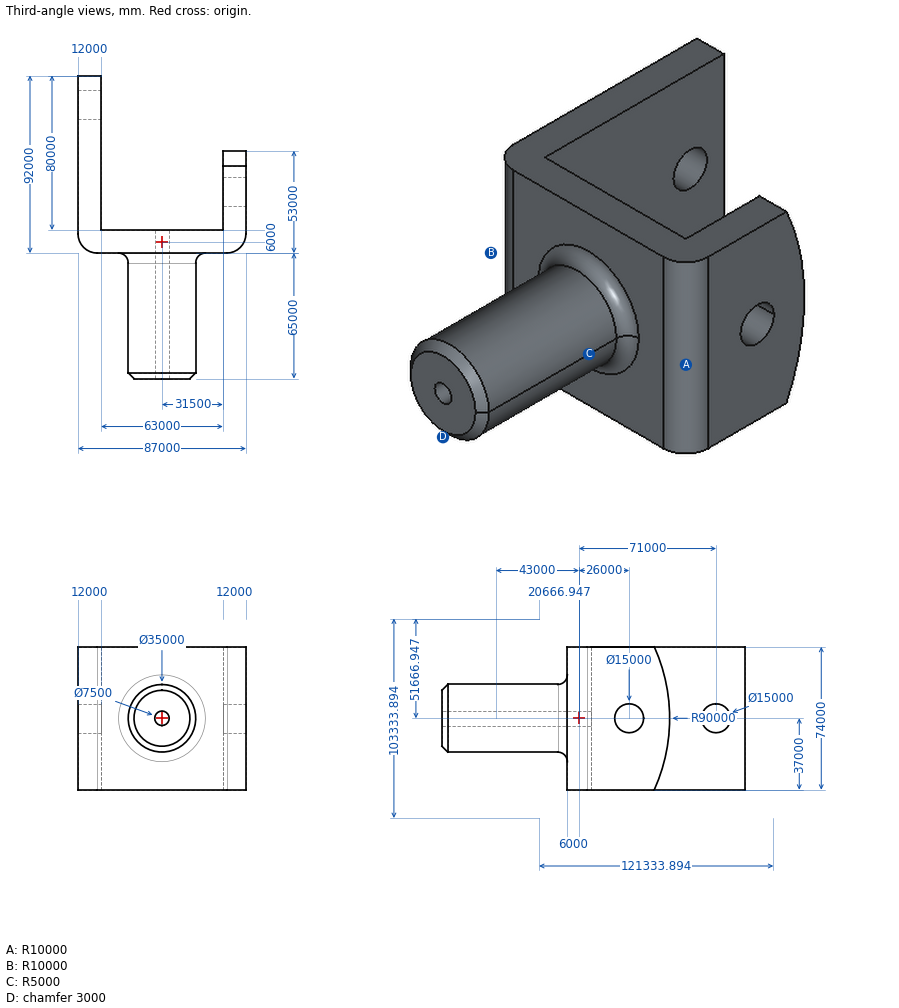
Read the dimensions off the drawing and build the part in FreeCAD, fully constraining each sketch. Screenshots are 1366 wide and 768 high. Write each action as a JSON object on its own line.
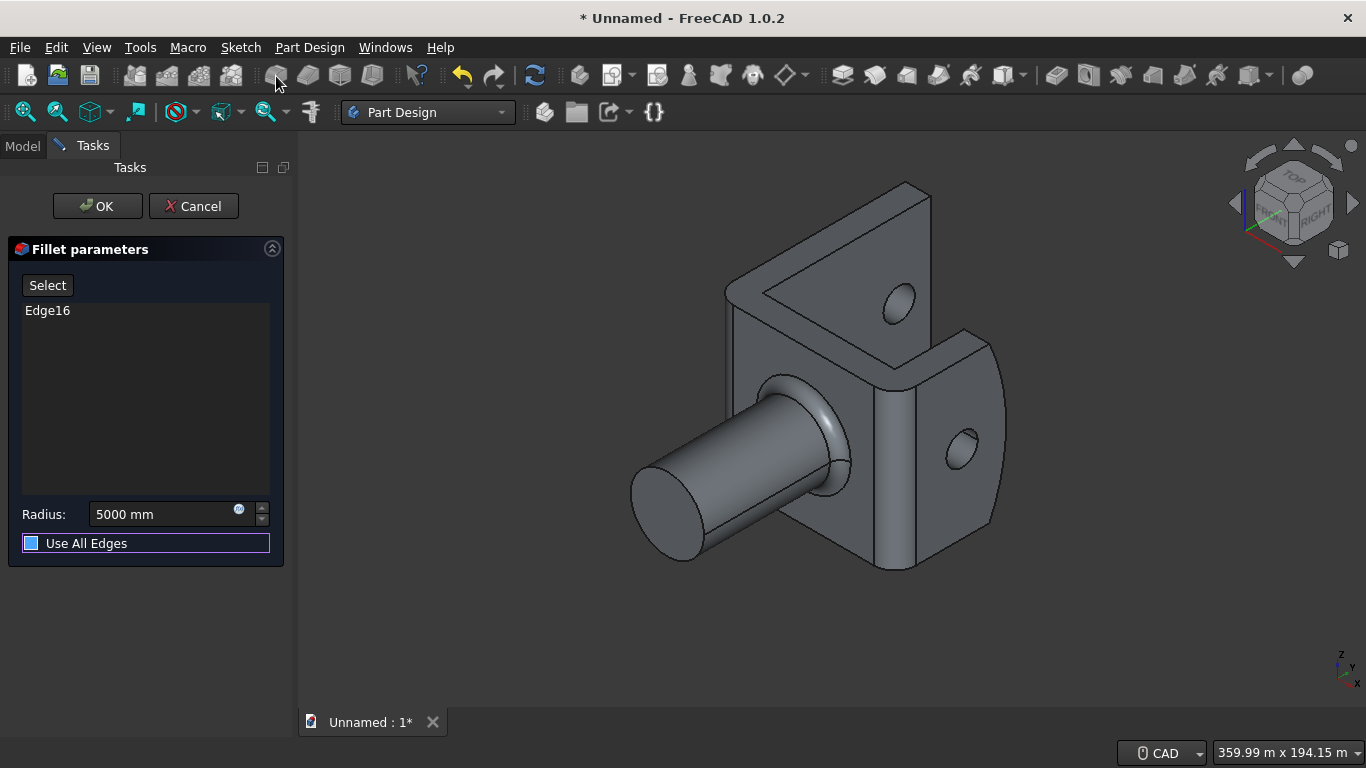
{"action": "left_click", "coordinate": [98, 206]}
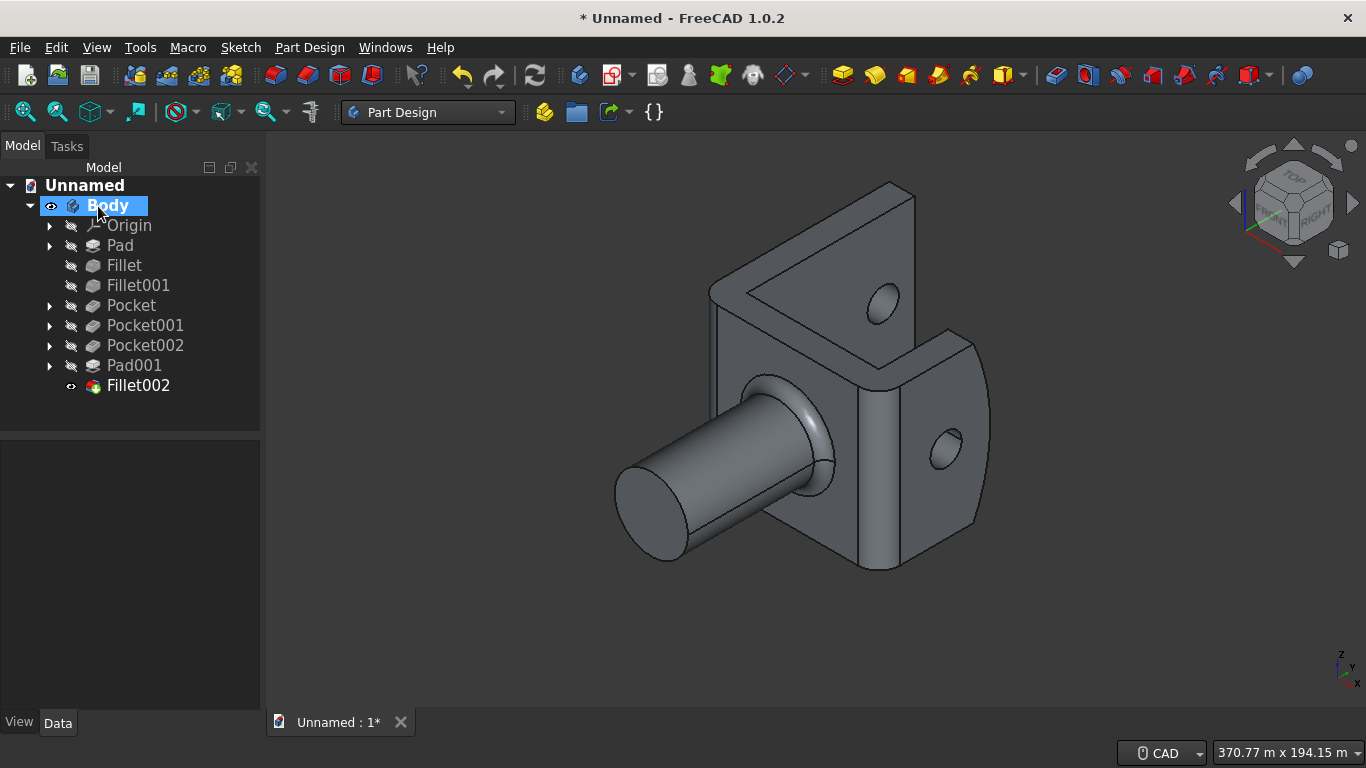
{"action": "left_click", "coordinate": [640, 466]}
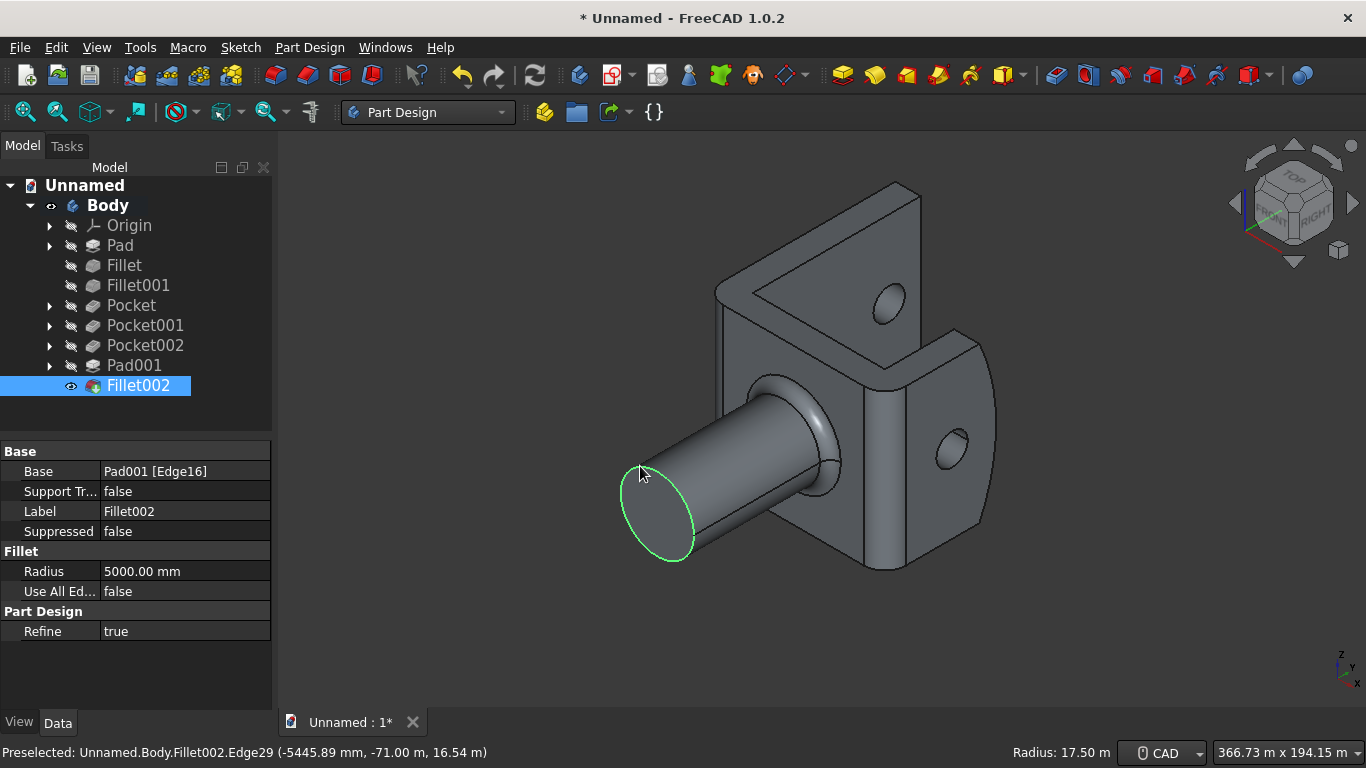
{"action": "left_click", "coordinate": [308, 76]}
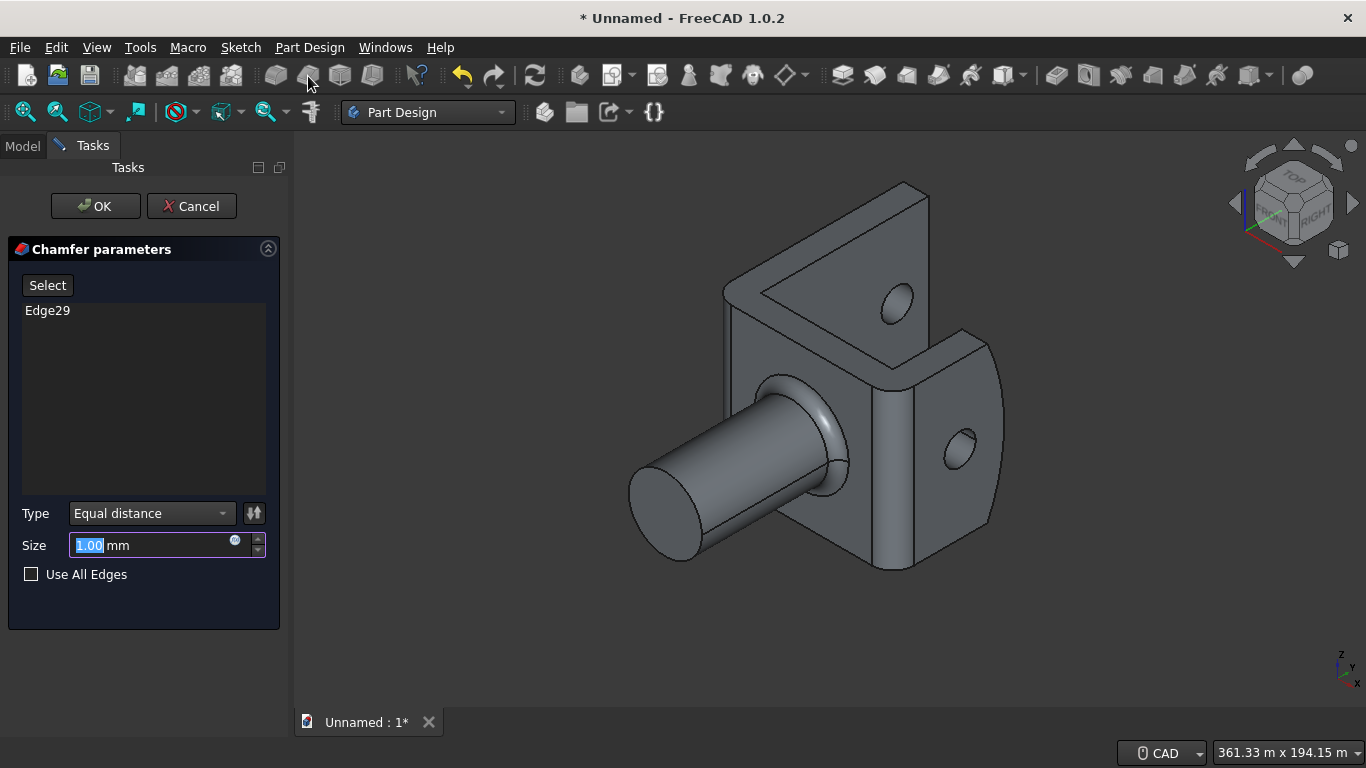
{"action": "type", "text": "3000"}
{"action": "key", "text": "Tab"}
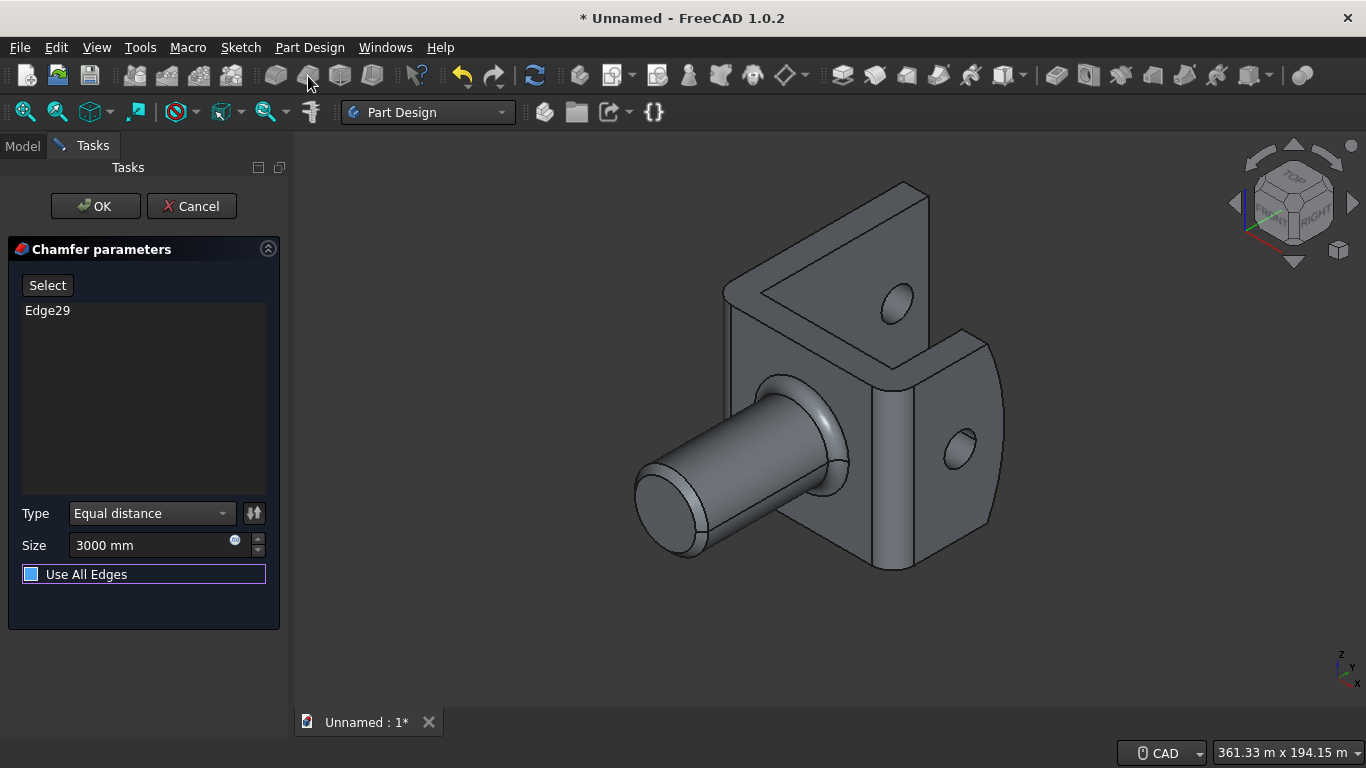
{"action": "left_click", "coordinate": [96, 206]}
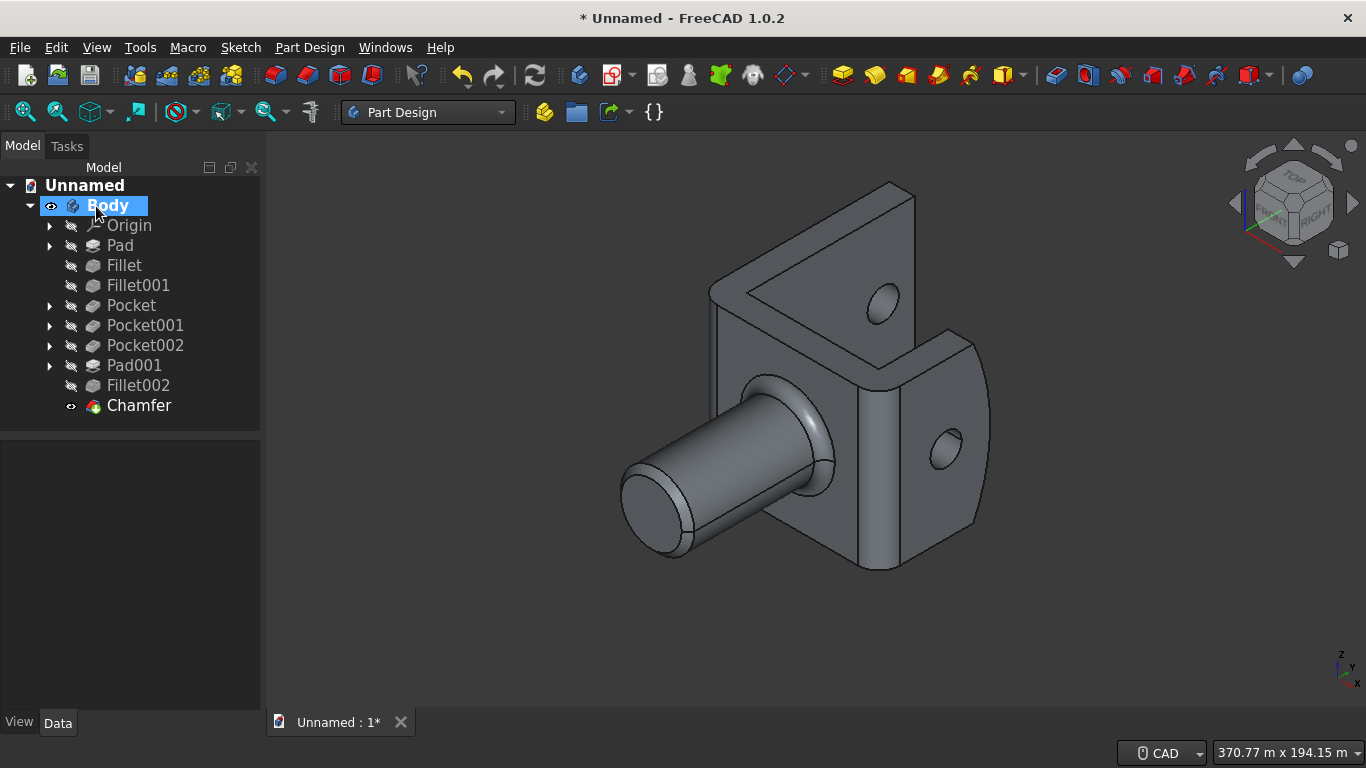
{"action": "left_click", "coordinate": [651, 513]}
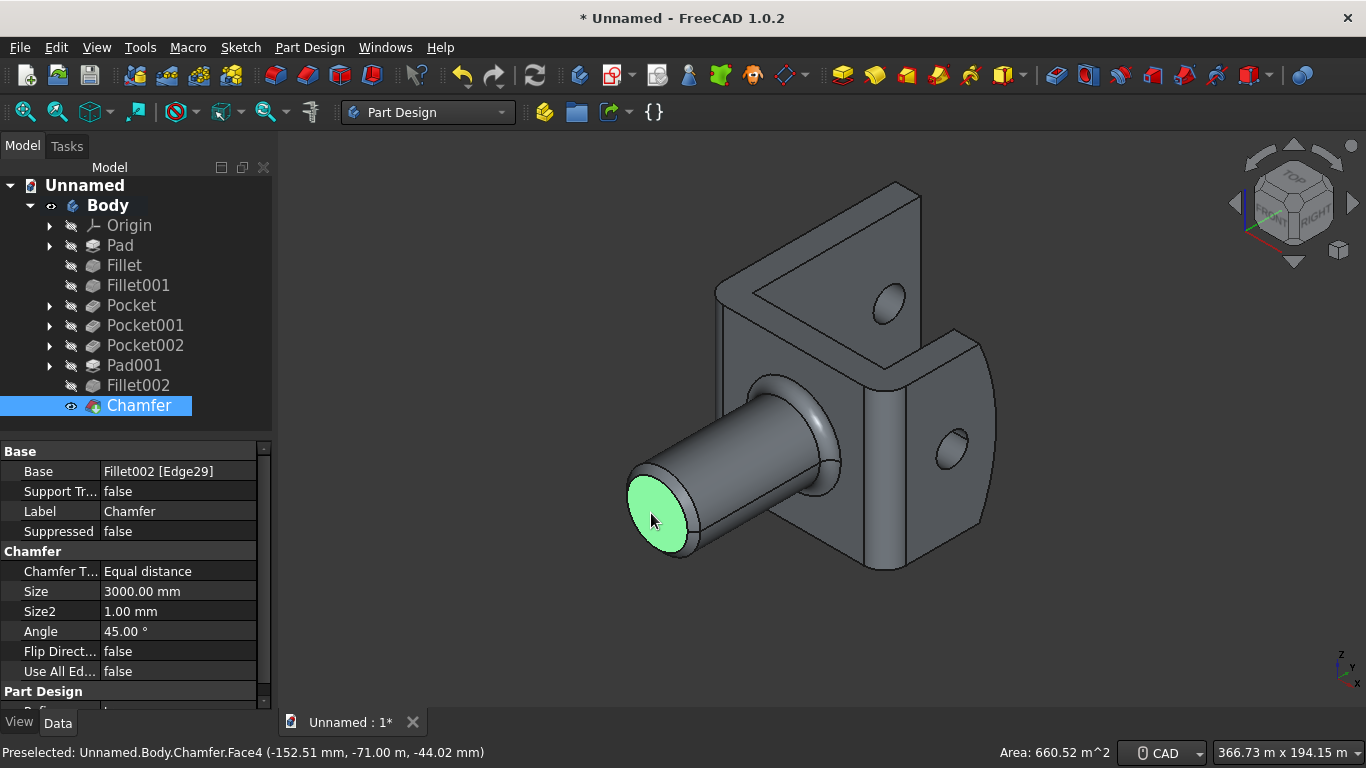
{"action": "left_click", "coordinate": [612, 76]}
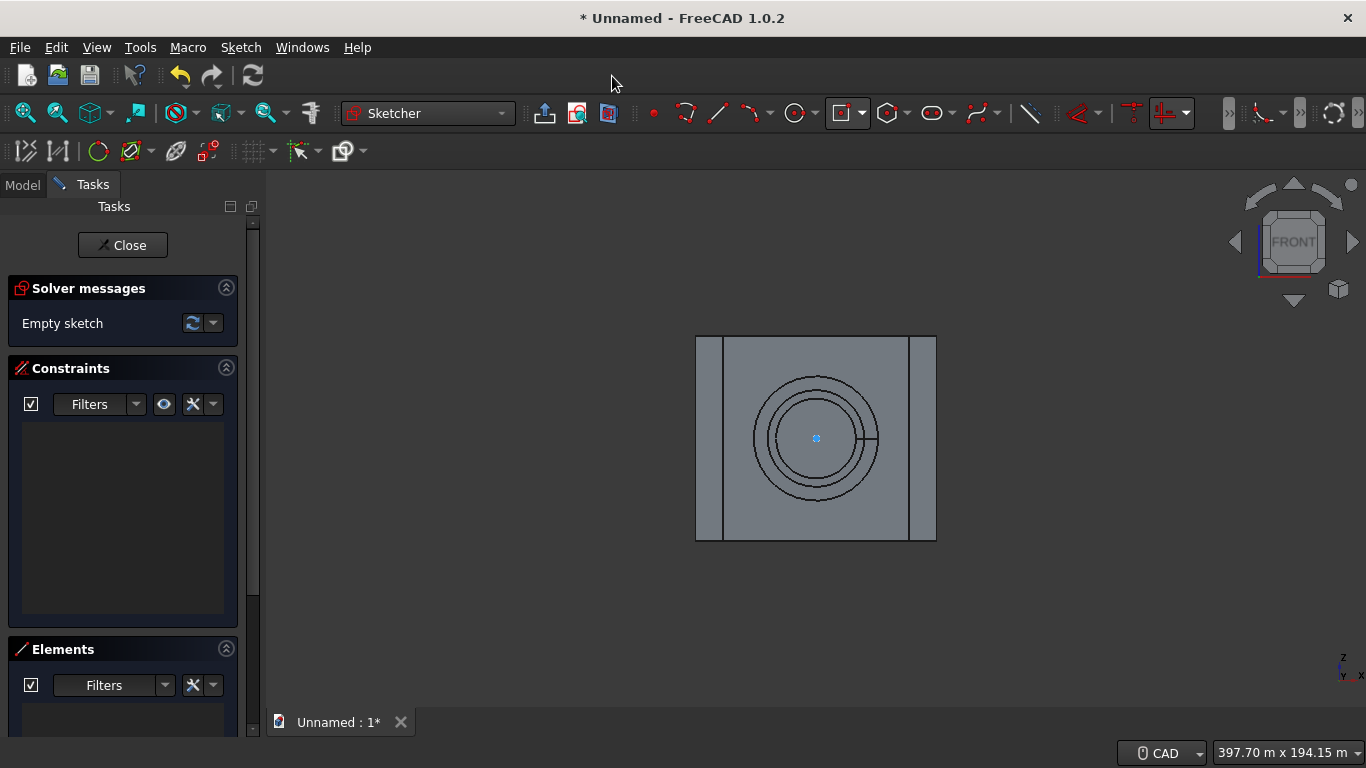
{"action": "scroll", "coordinate": [820, 439], "scroll_direction": "up", "scroll_amount": 14}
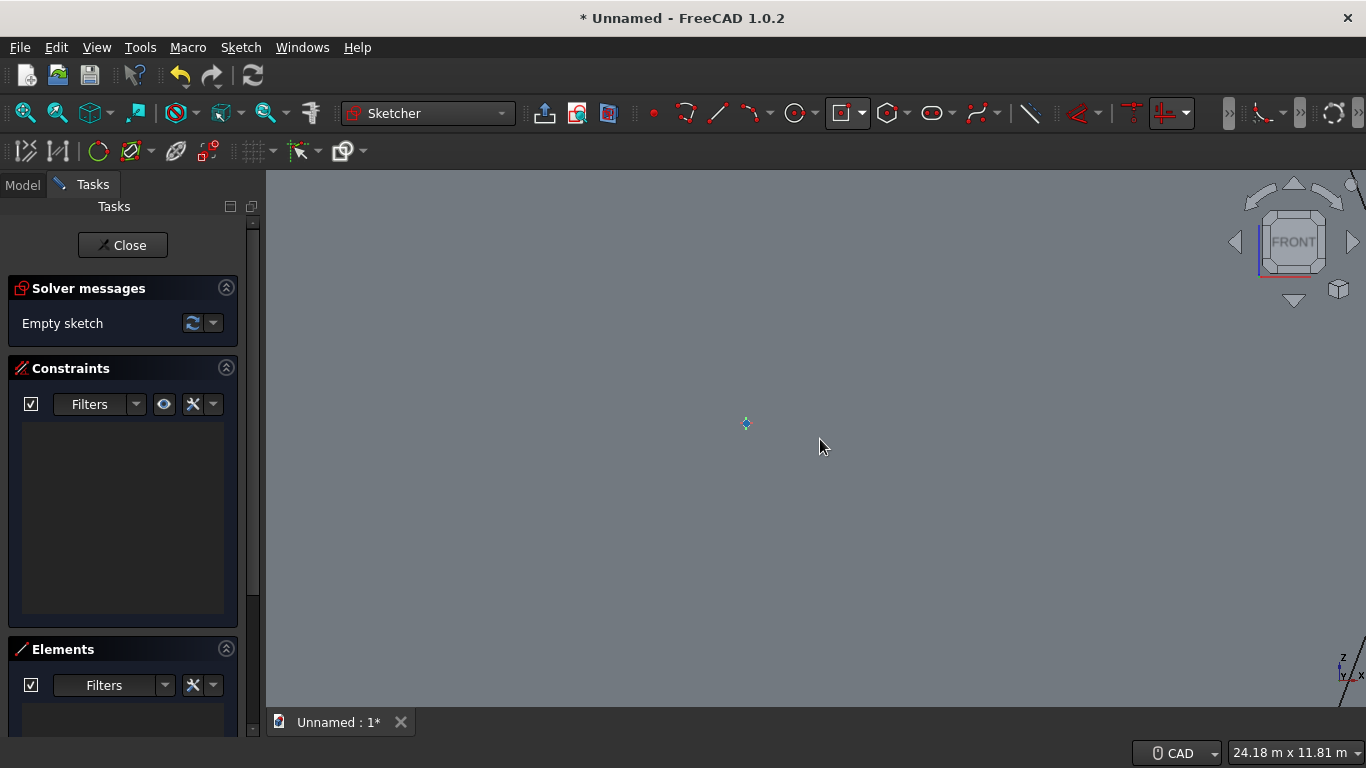
{"action": "left_click", "coordinate": [796, 114]}